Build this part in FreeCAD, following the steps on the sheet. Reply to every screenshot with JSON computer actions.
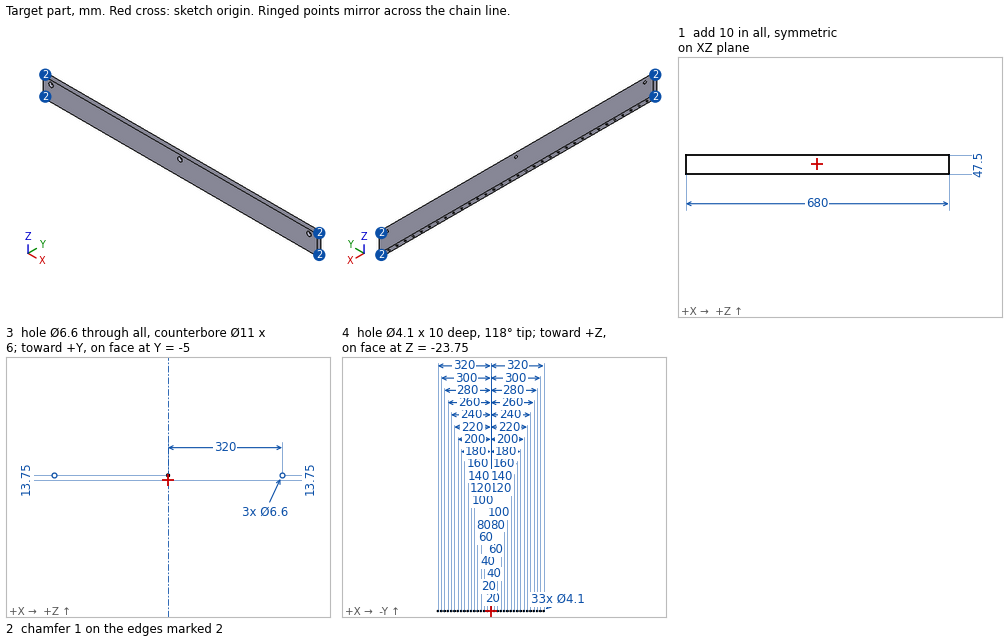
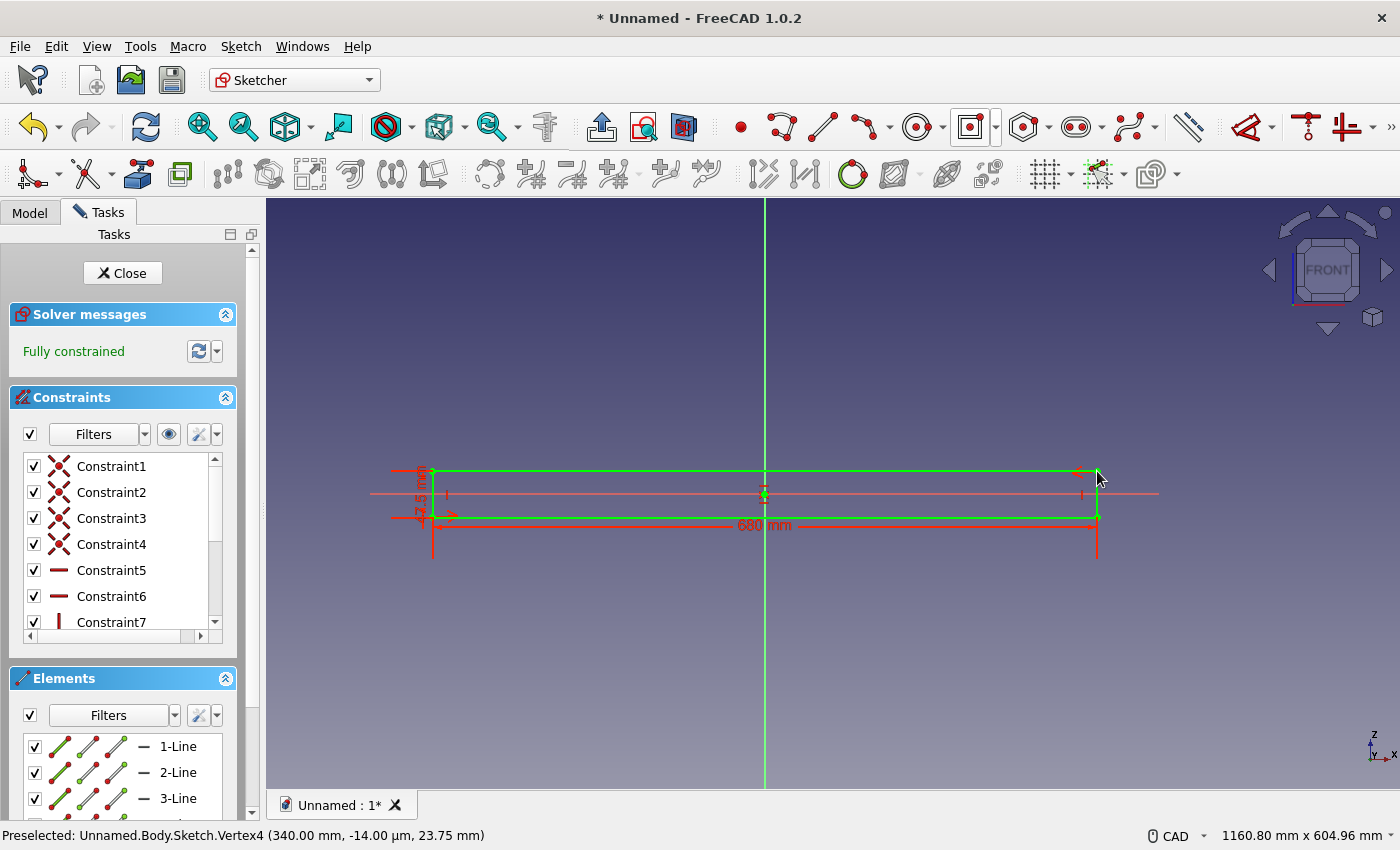
{"action": "left_click", "coordinate": [123, 273]}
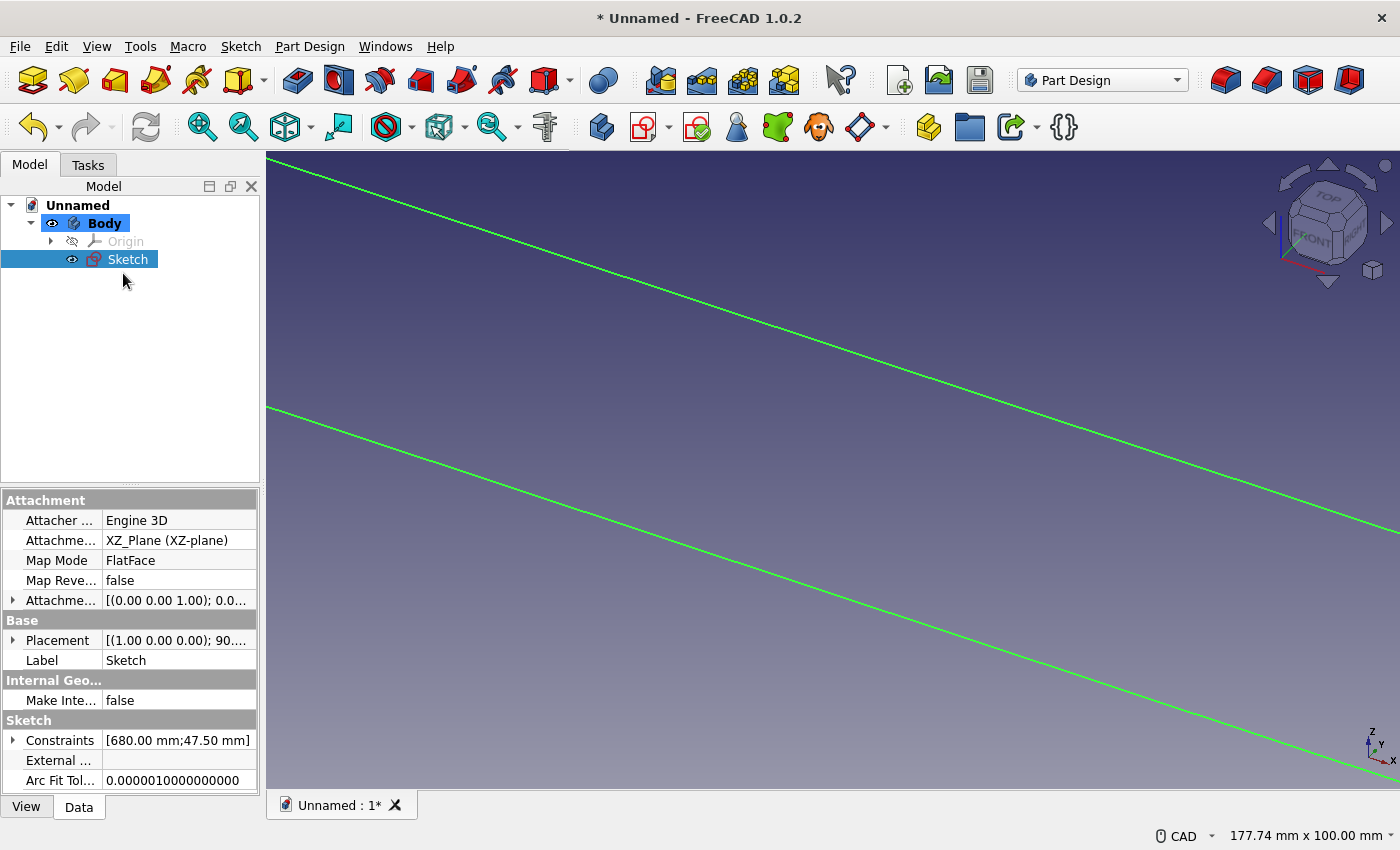
{"action": "left_click", "coordinate": [33, 80]}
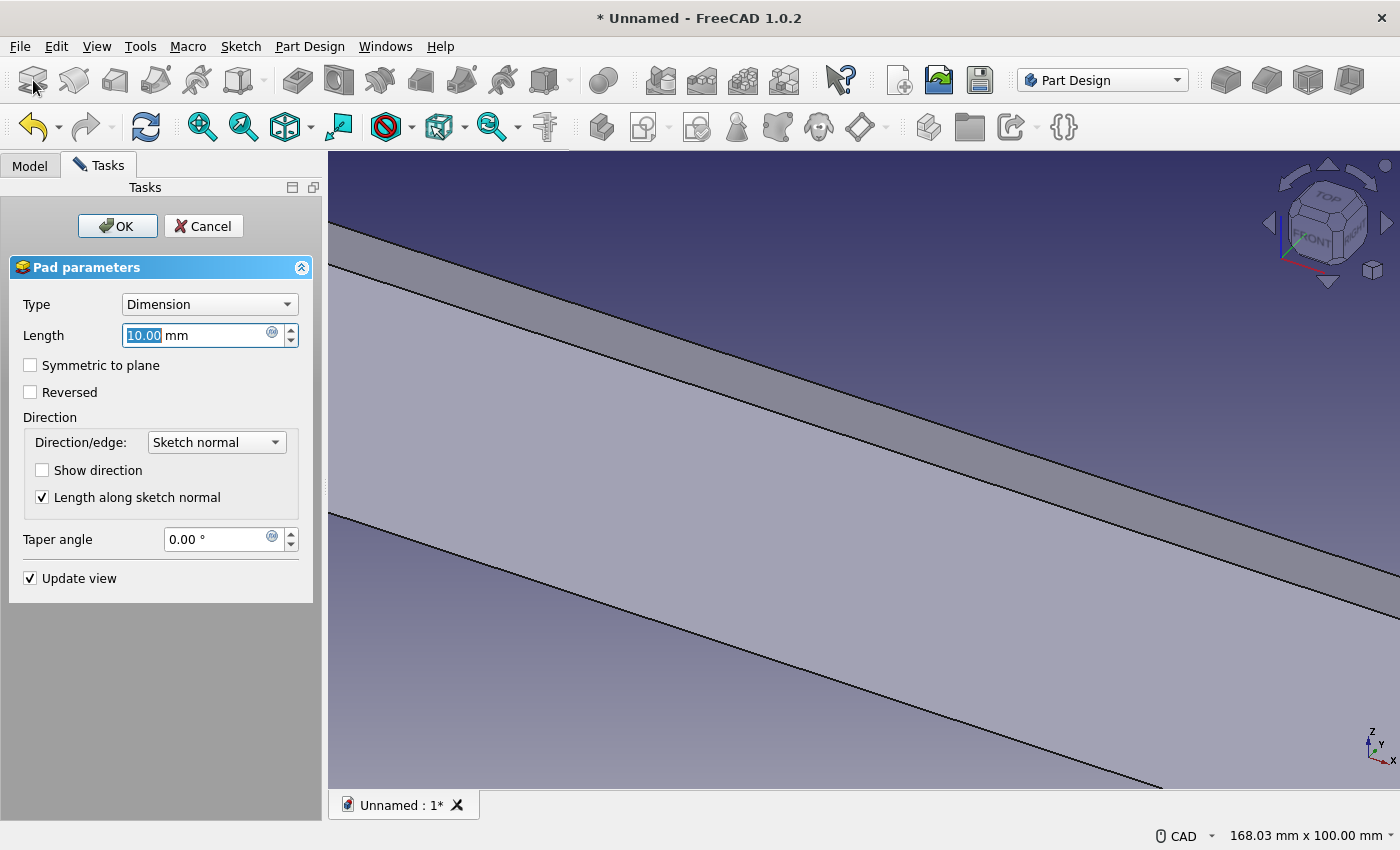
{"action": "type", "text": "10"}
{"action": "key", "text": "Tab"}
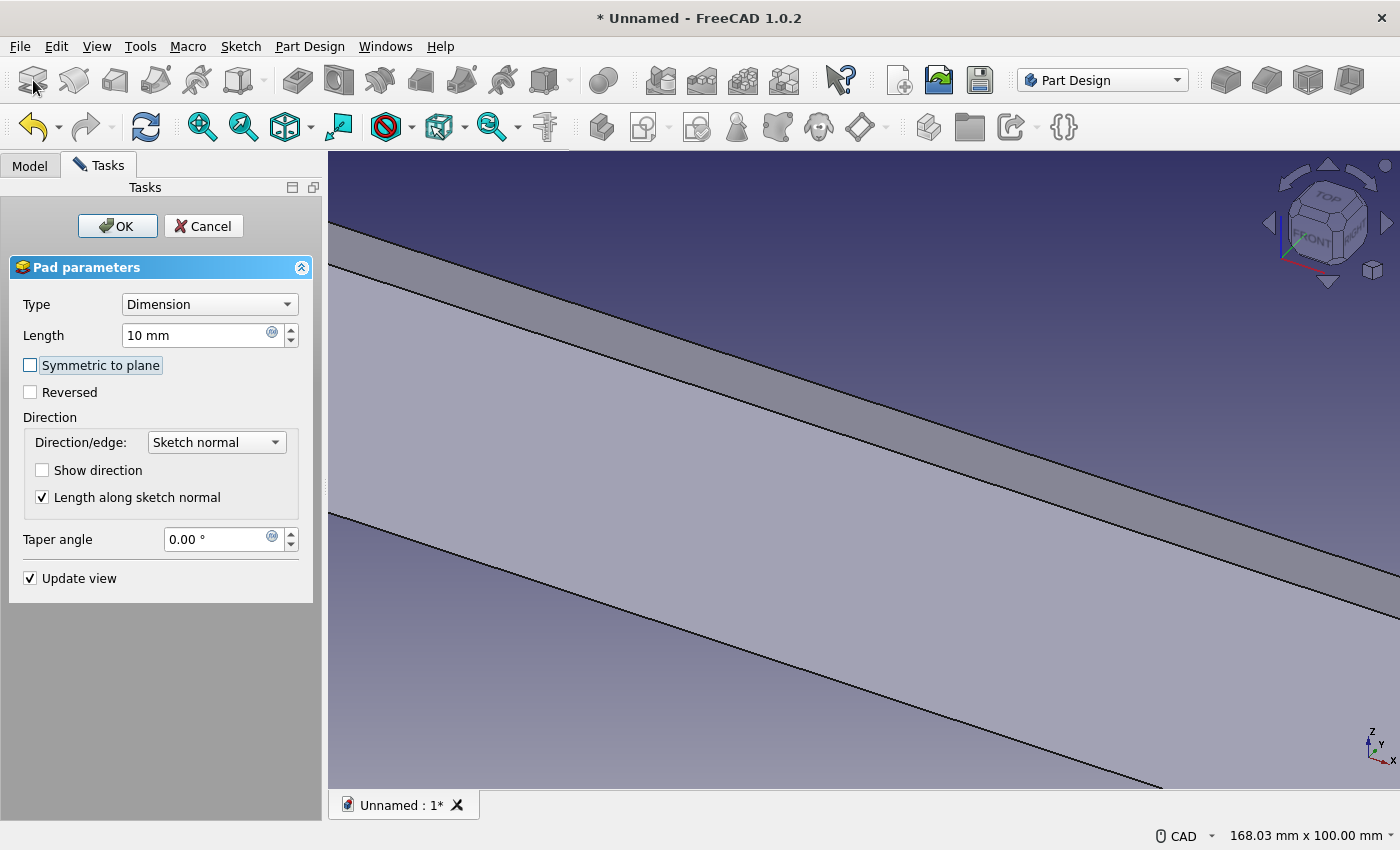
{"action": "left_click", "coordinate": [31, 365]}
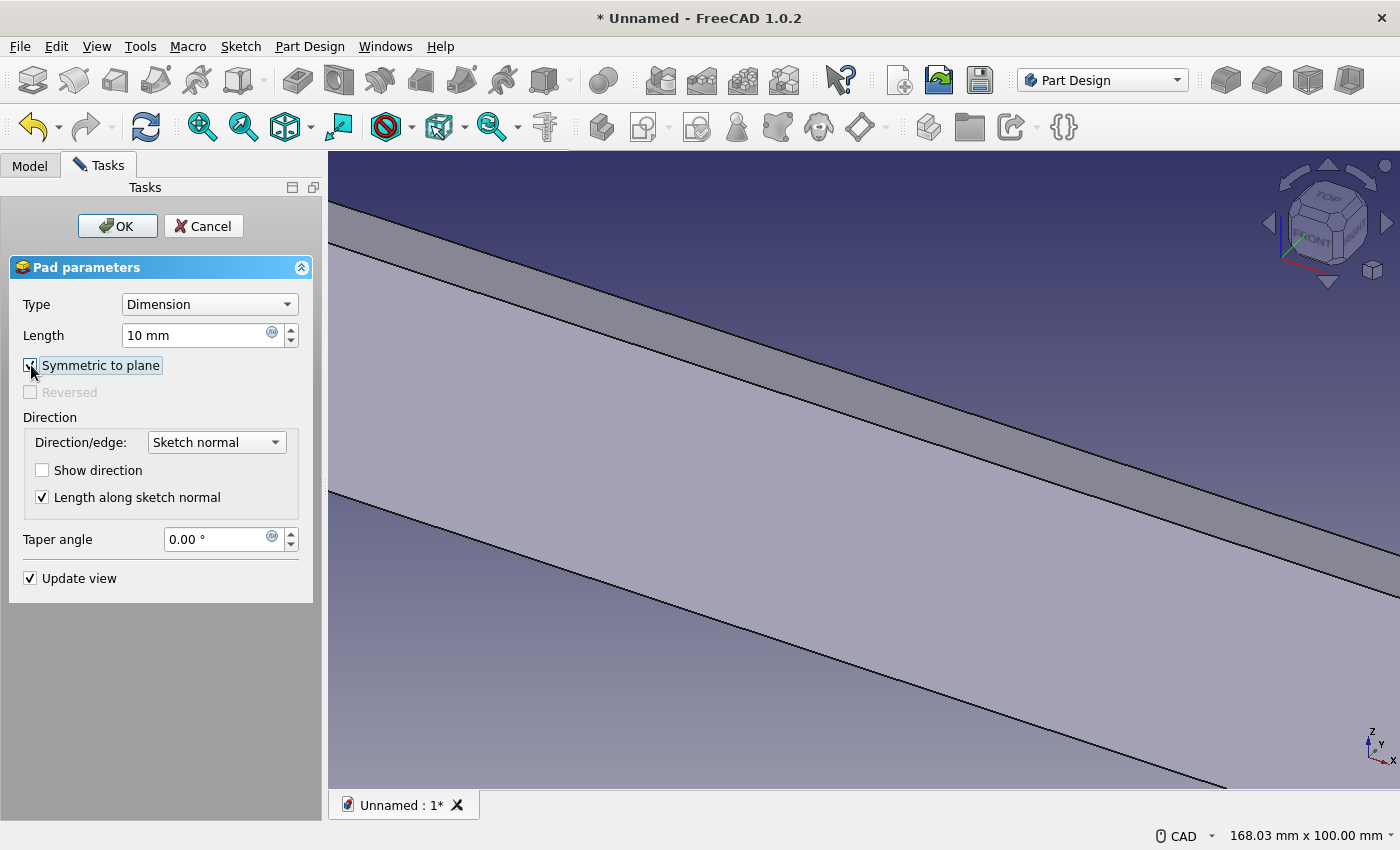
{"action": "left_click", "coordinate": [118, 226]}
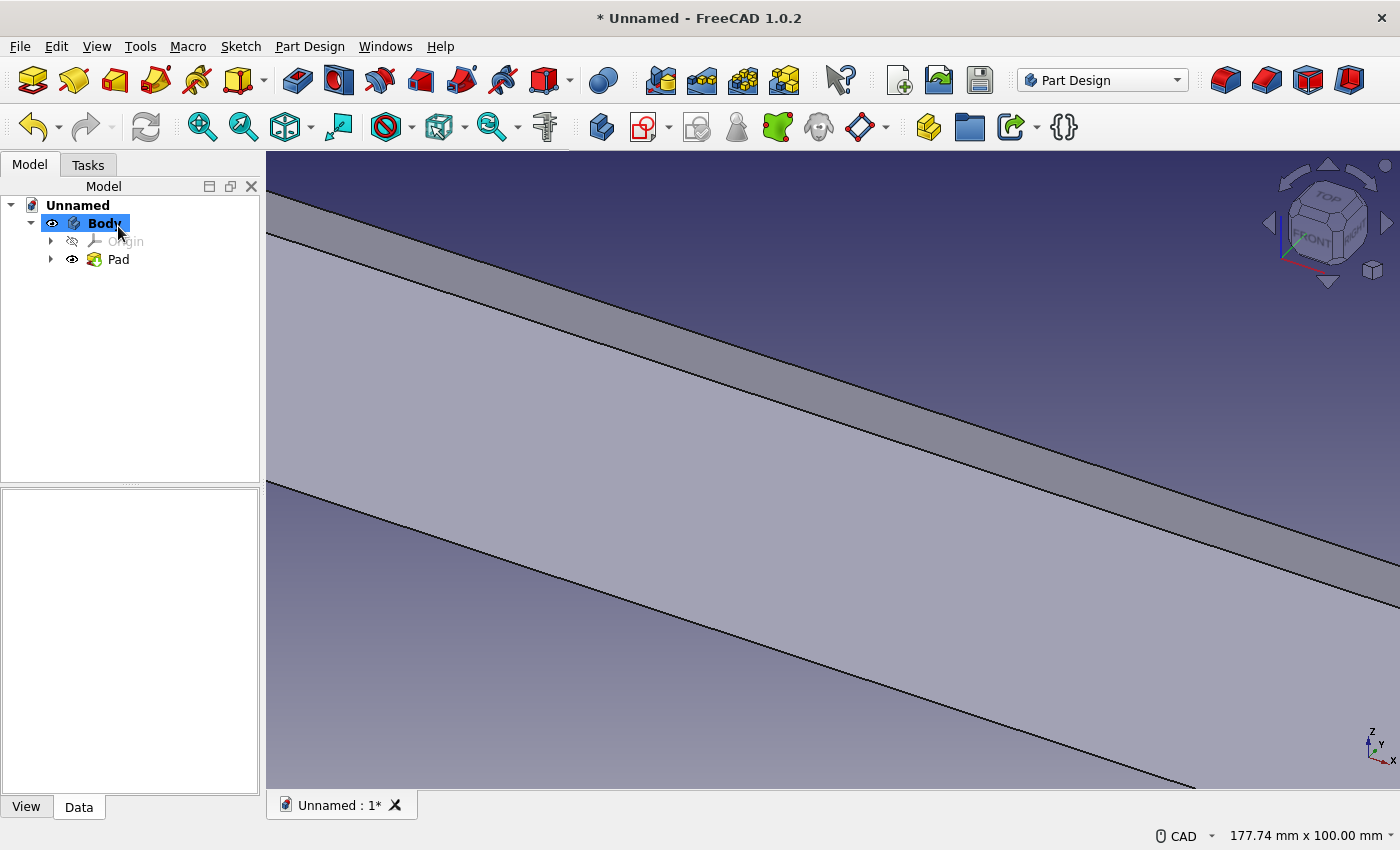
{"action": "left_click", "coordinate": [203, 128]}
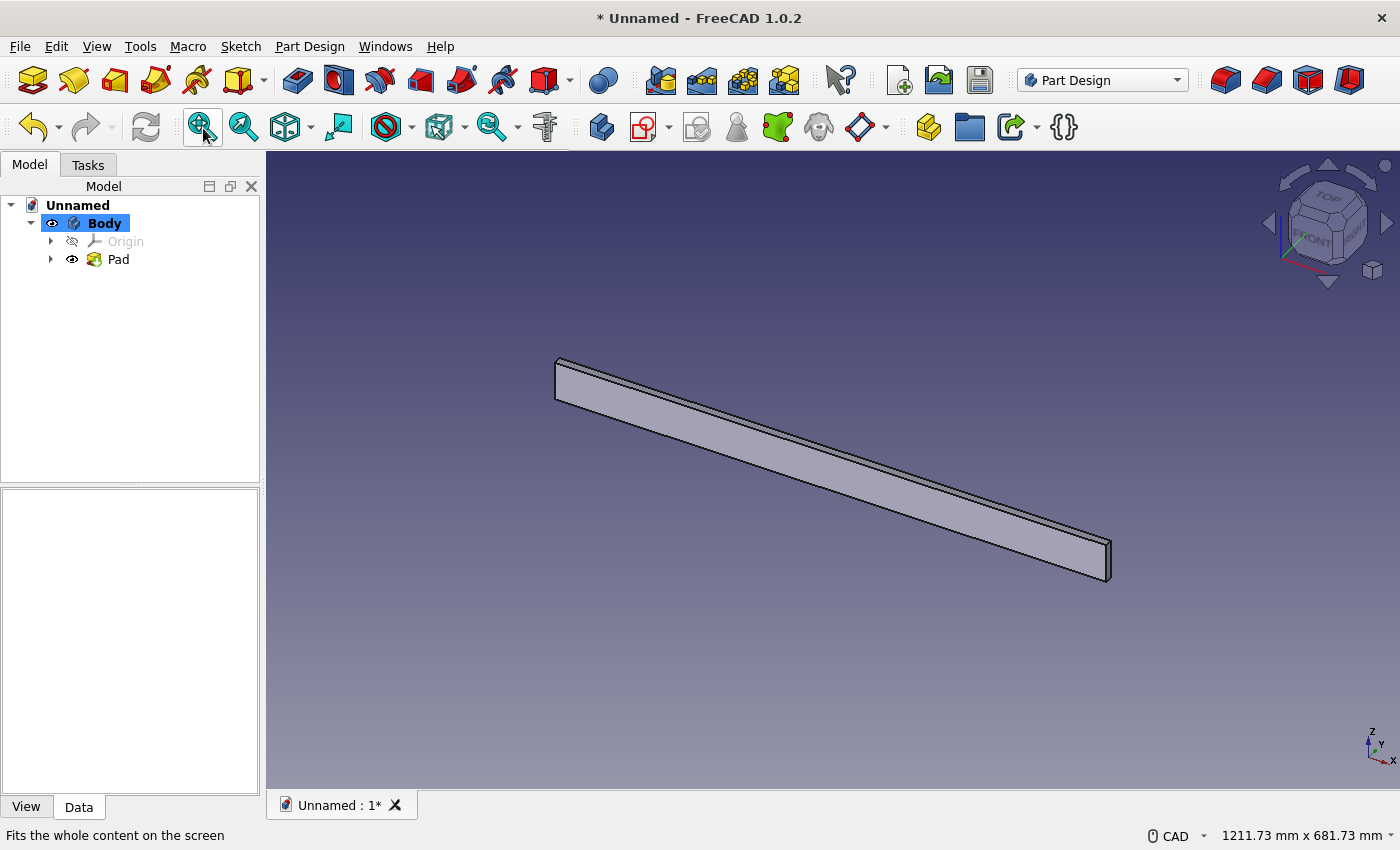
{"action": "scroll", "coordinate": [1109, 542], "scroll_direction": "up", "scroll_amount": 8}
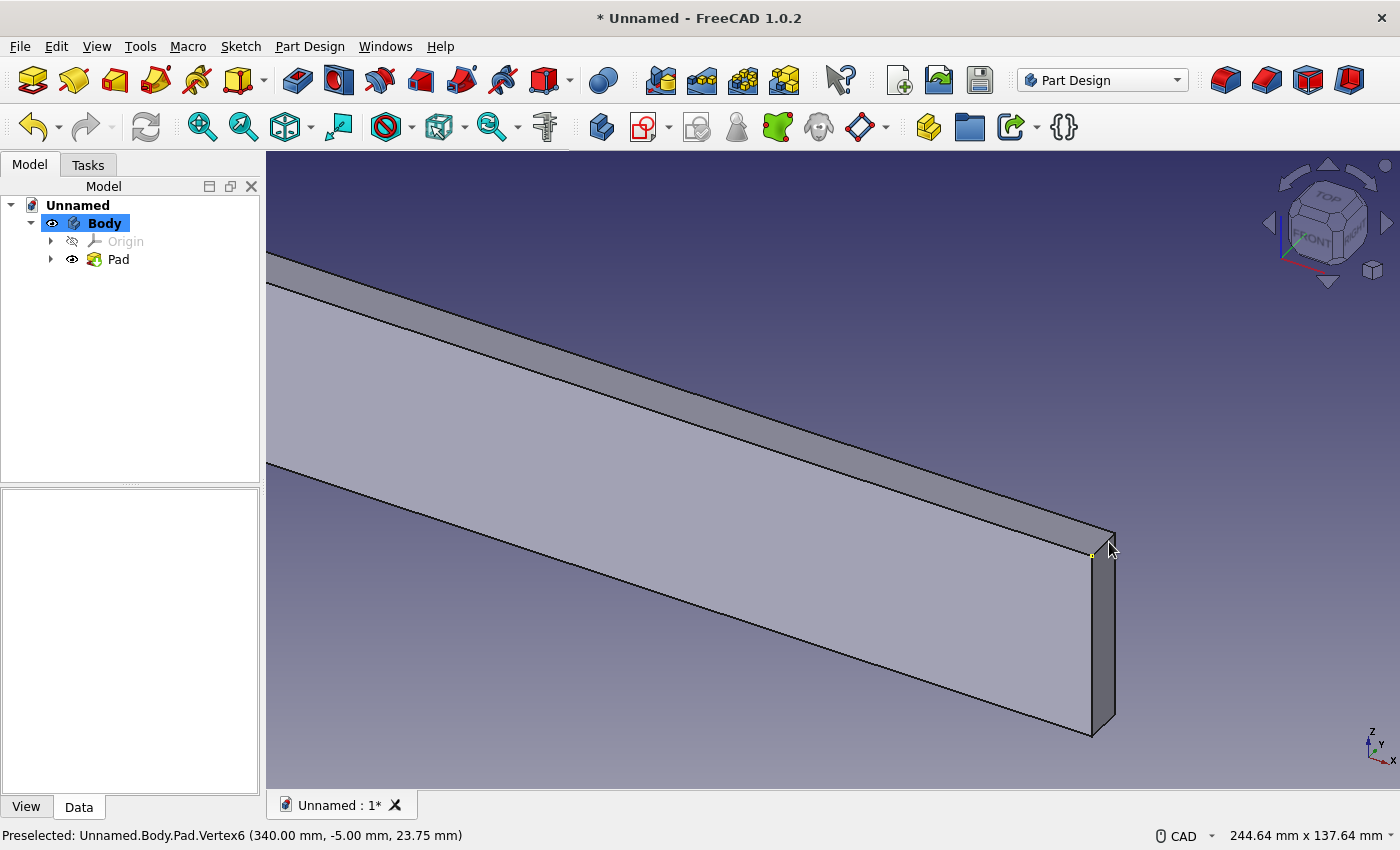
{"action": "left_click", "coordinate": [1104, 544]}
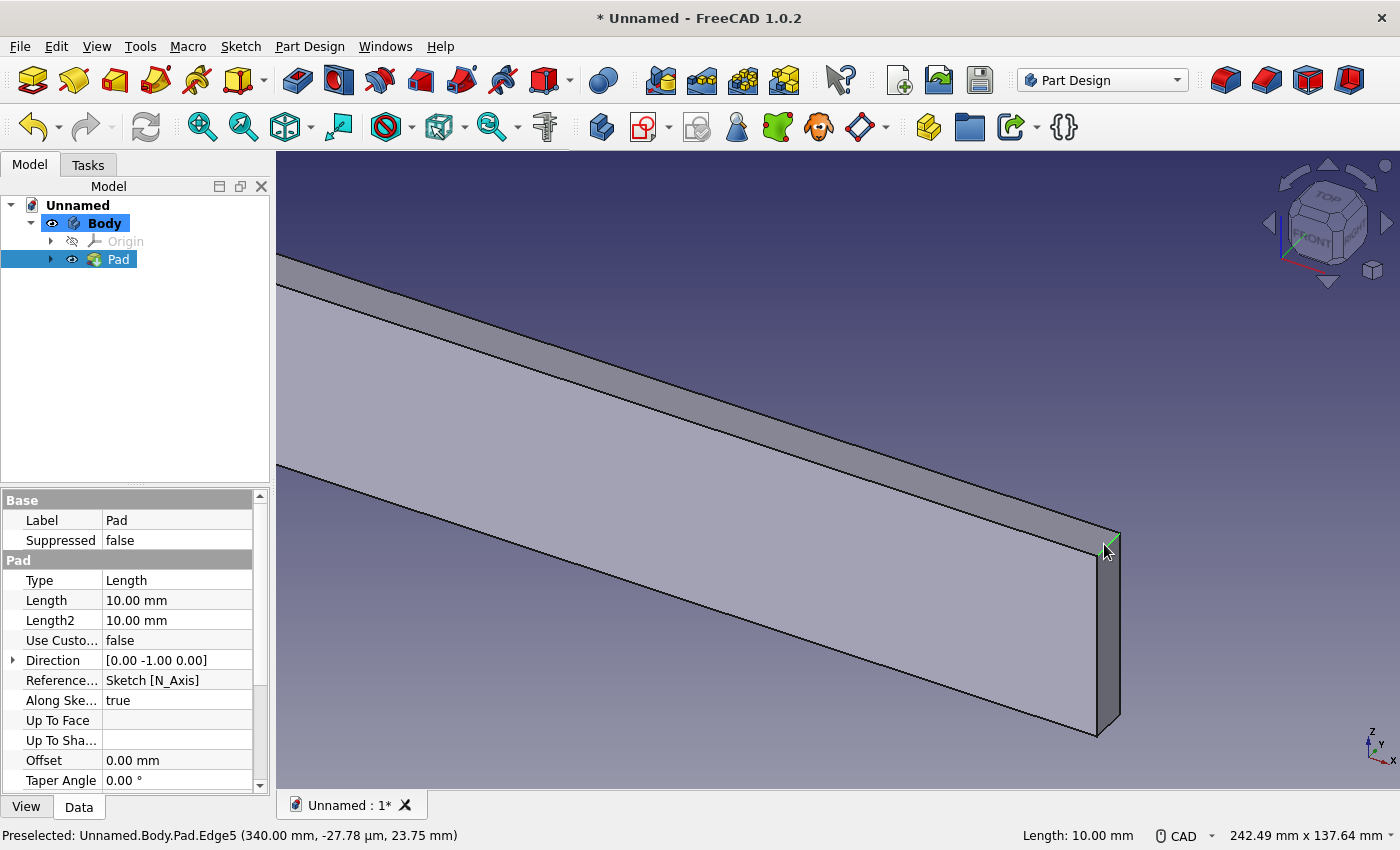
{"action": "left_click", "coordinate": [203, 128]}